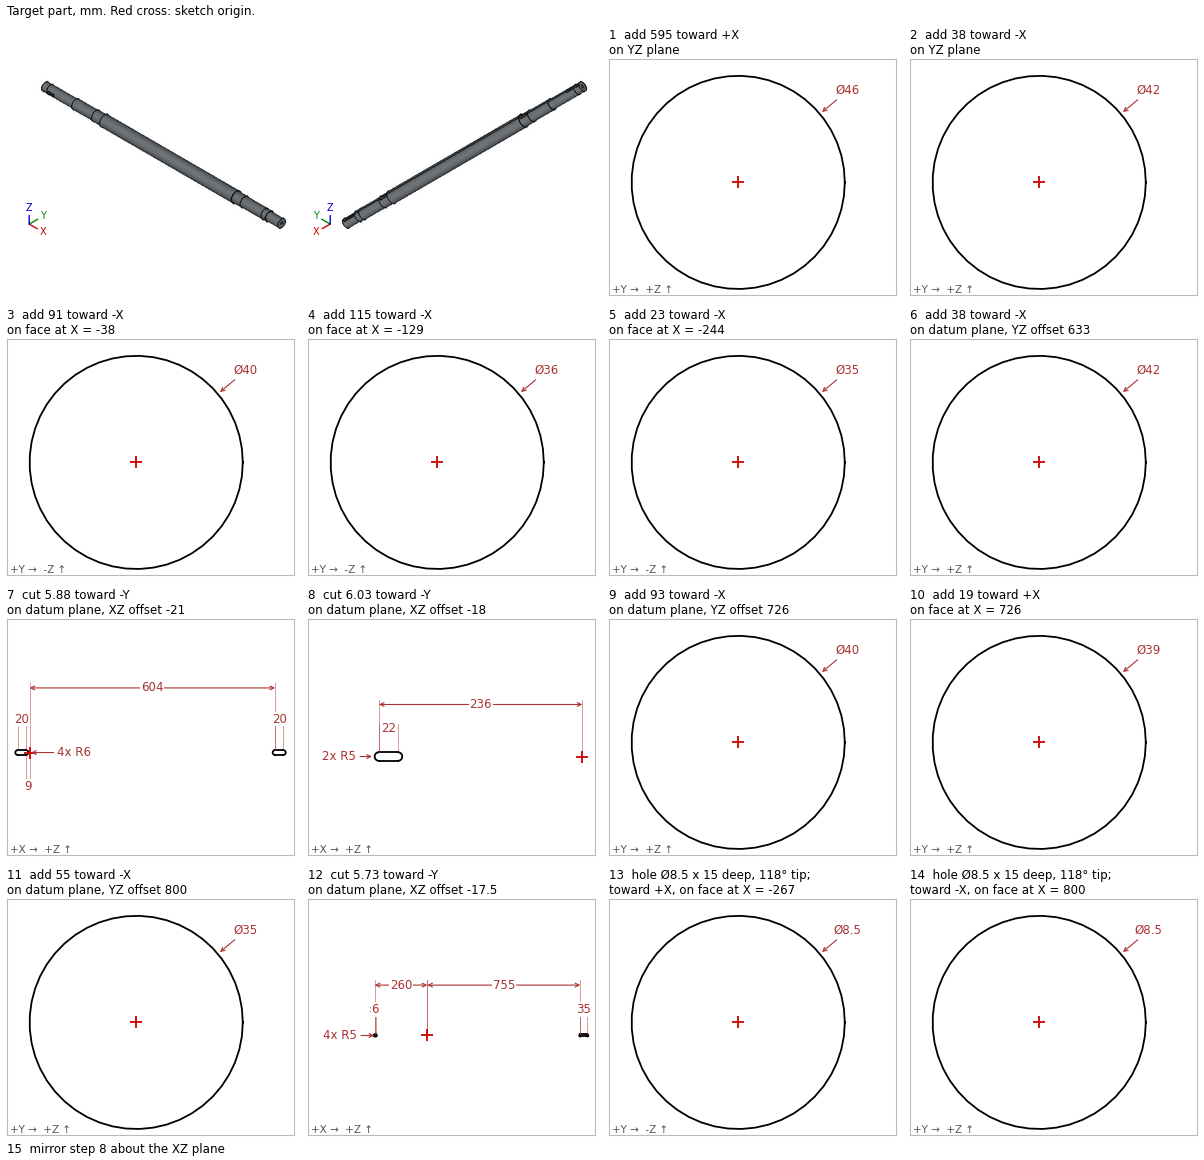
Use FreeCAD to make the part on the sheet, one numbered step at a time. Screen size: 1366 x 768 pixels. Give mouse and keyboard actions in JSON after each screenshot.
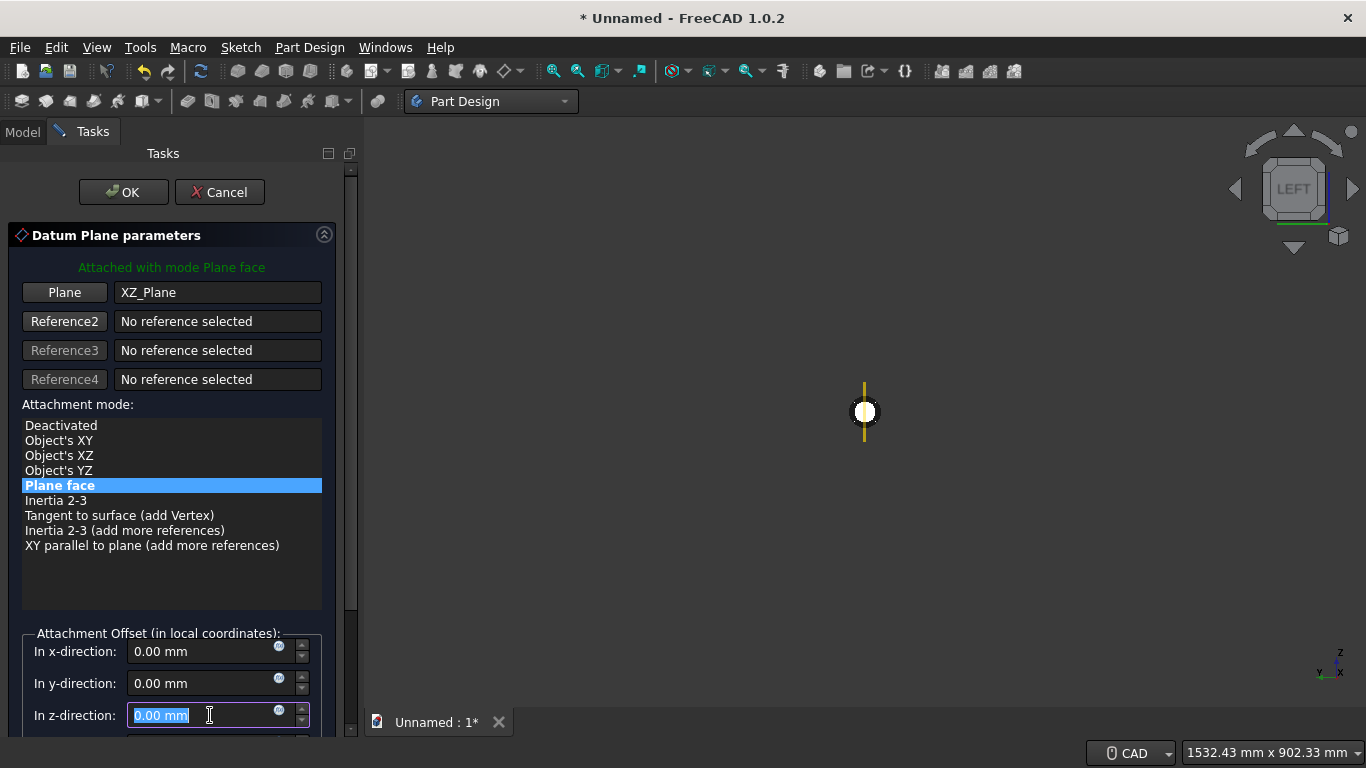
{"action": "type", "text": "-18"}
{"action": "key", "text": "Tab"}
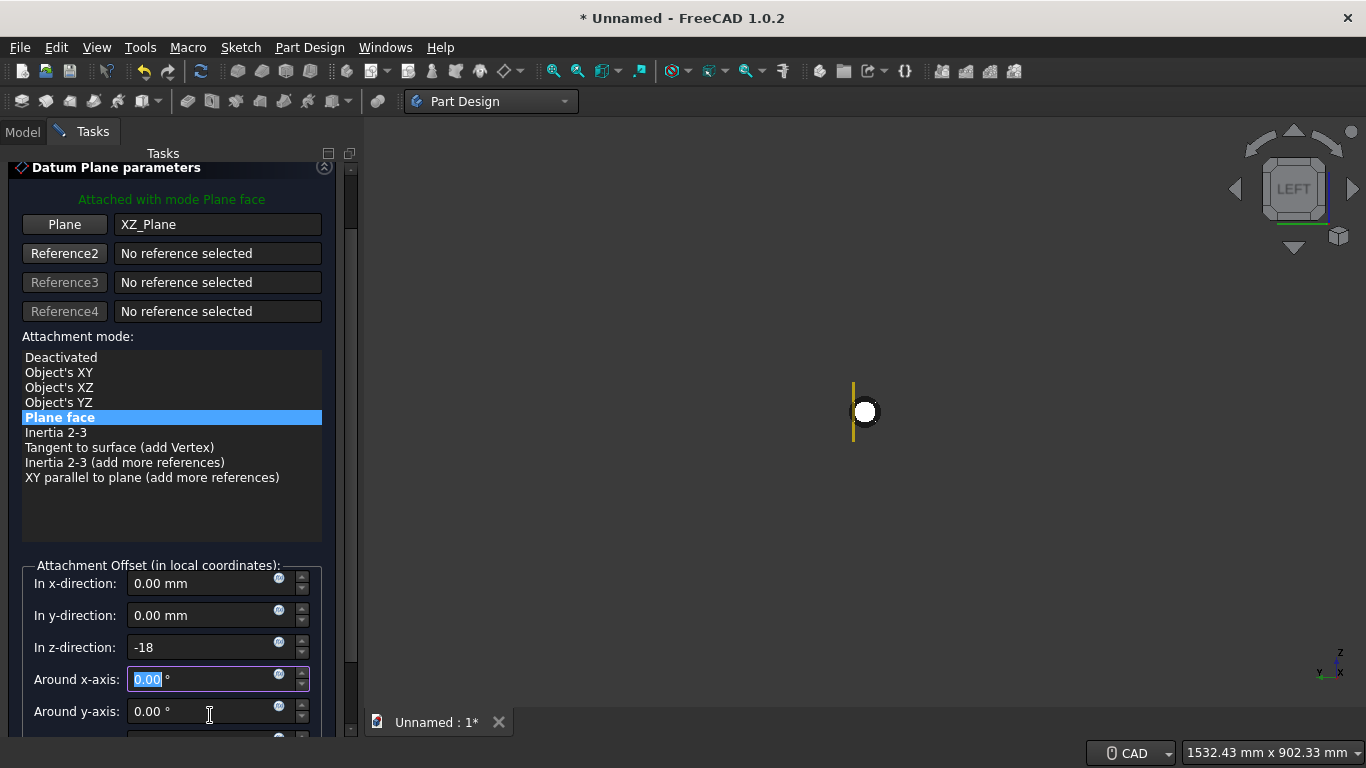
{"action": "scroll", "coordinate": [351, 450], "scroll_direction": "up", "scroll_amount": 2}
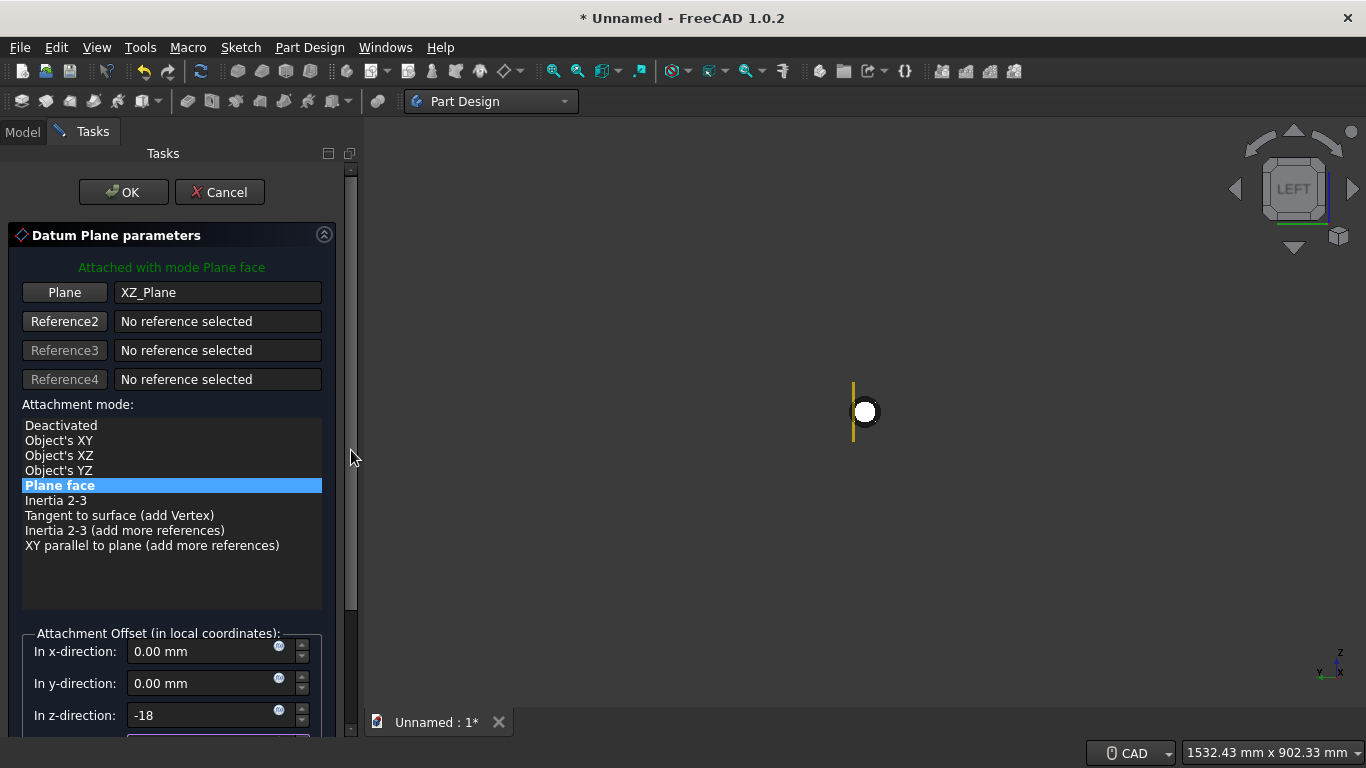
{"action": "left_click", "coordinate": [124, 192]}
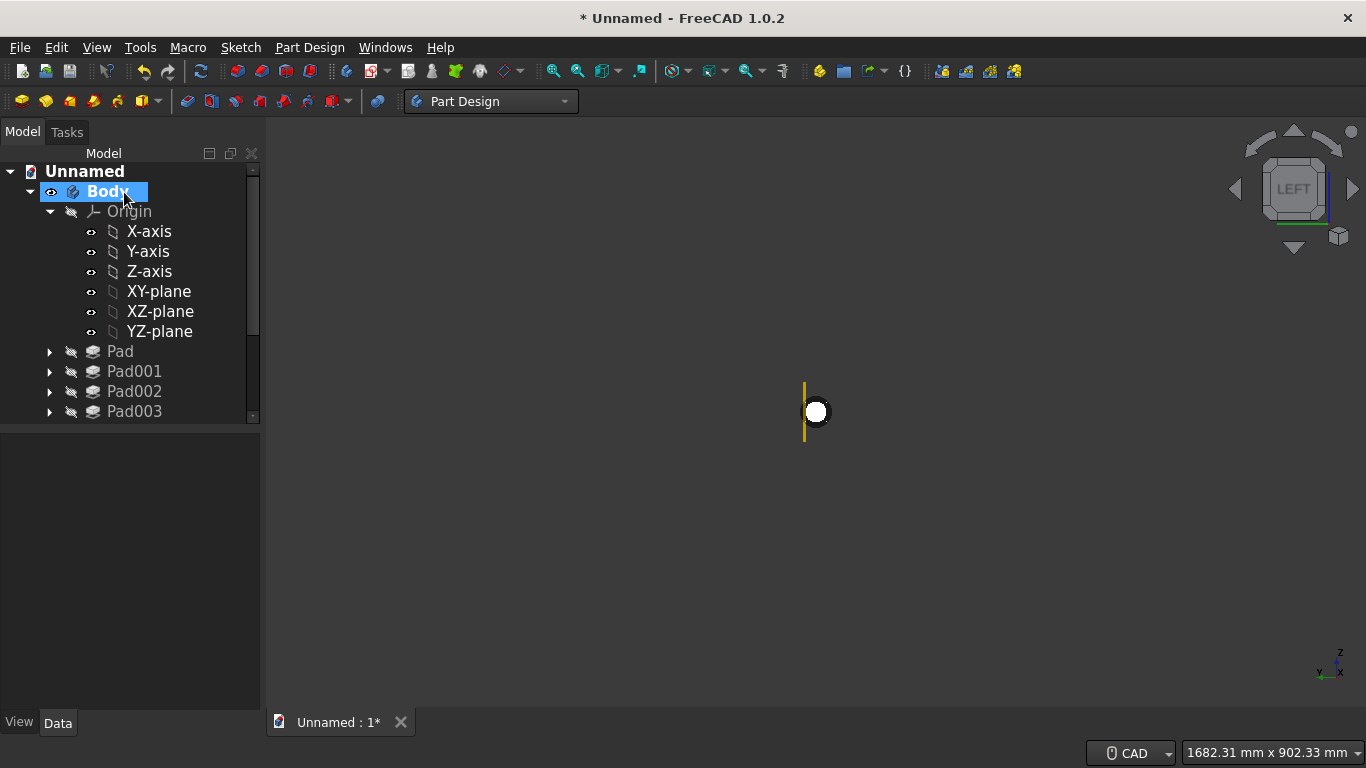
{"action": "scroll", "coordinate": [100, 287], "scroll_direction": "down", "scroll_amount": 3}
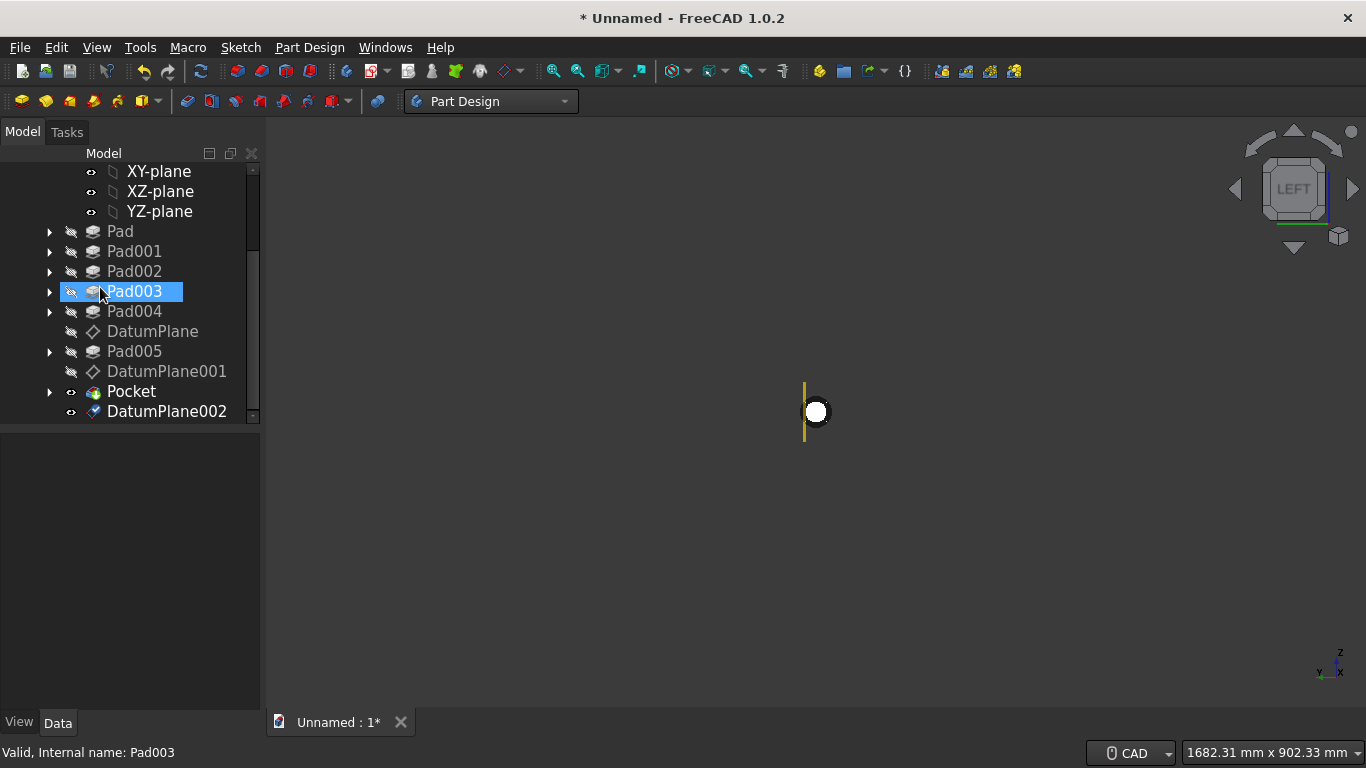
{"action": "left_click", "coordinate": [116, 412]}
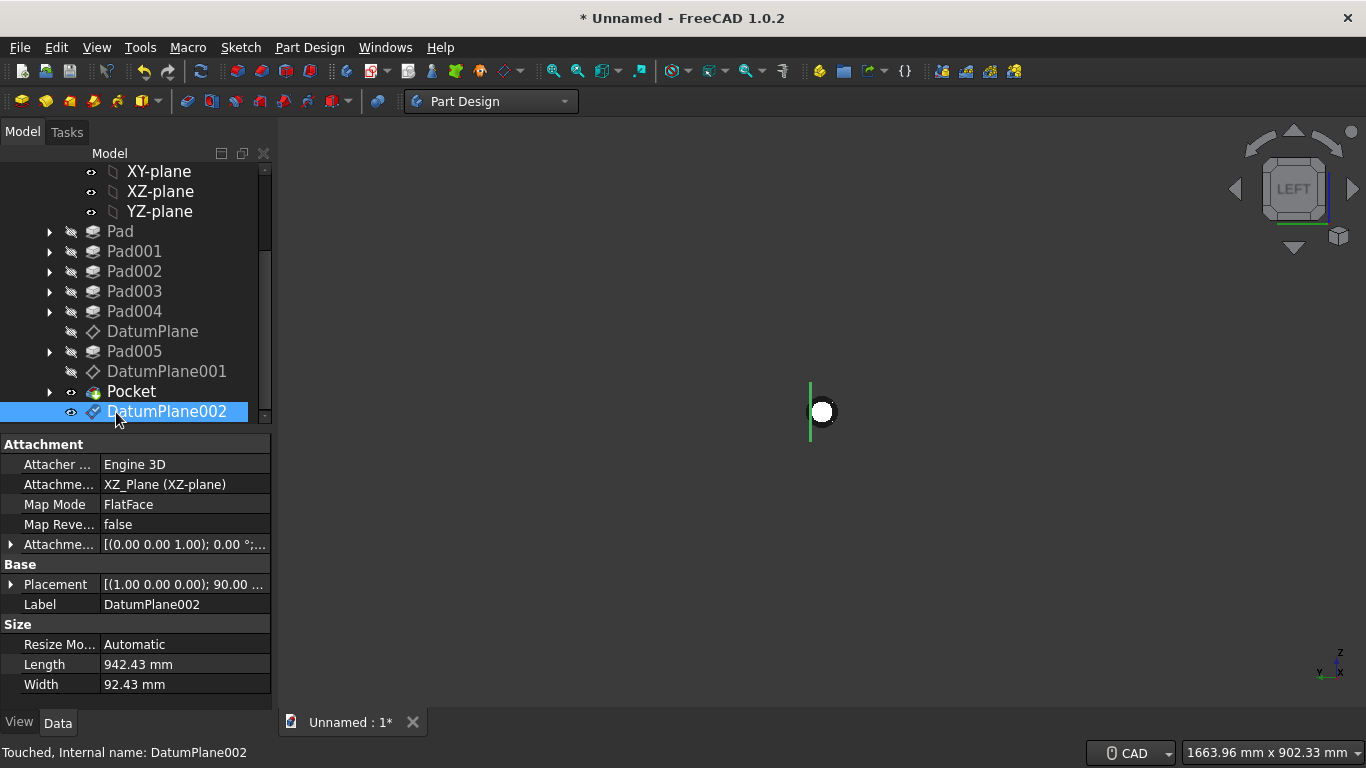
{"action": "left_click", "coordinate": [372, 72]}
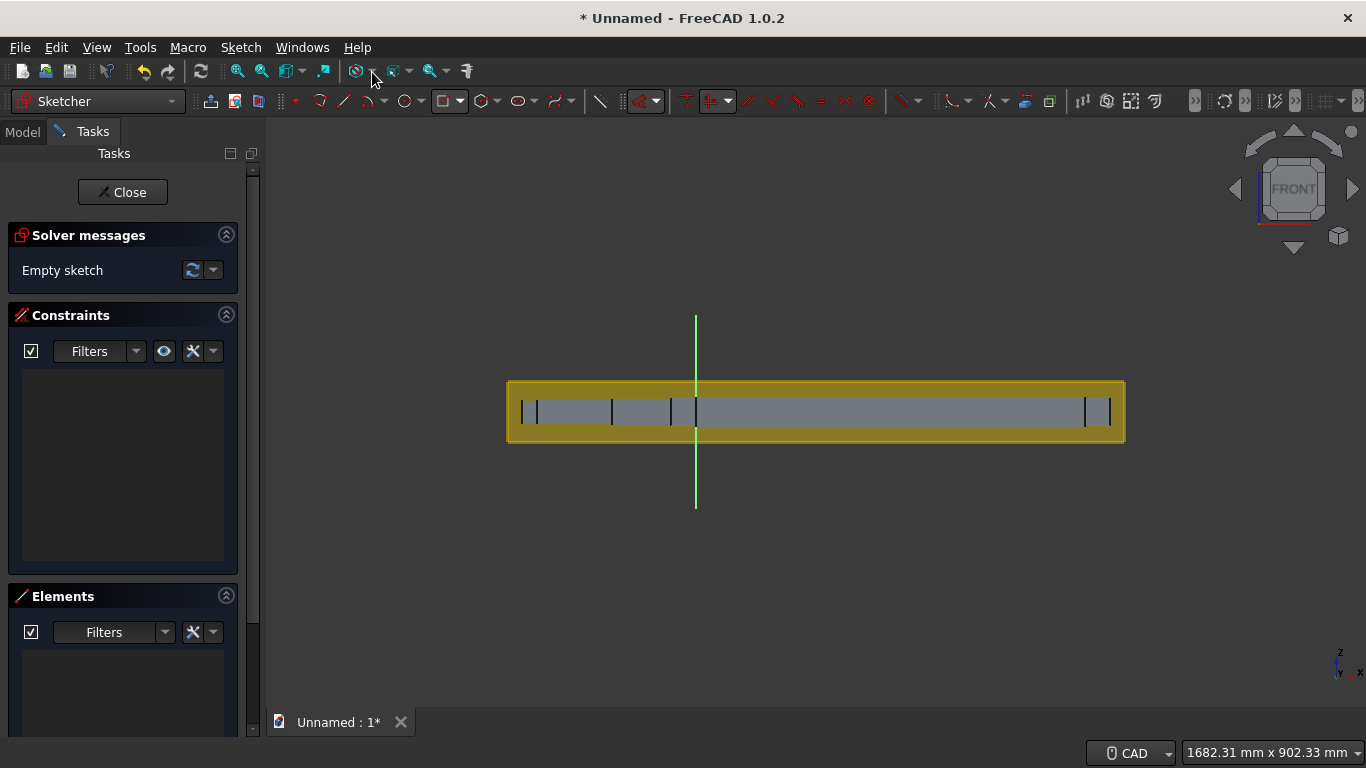
{"action": "key", "text": "q s"}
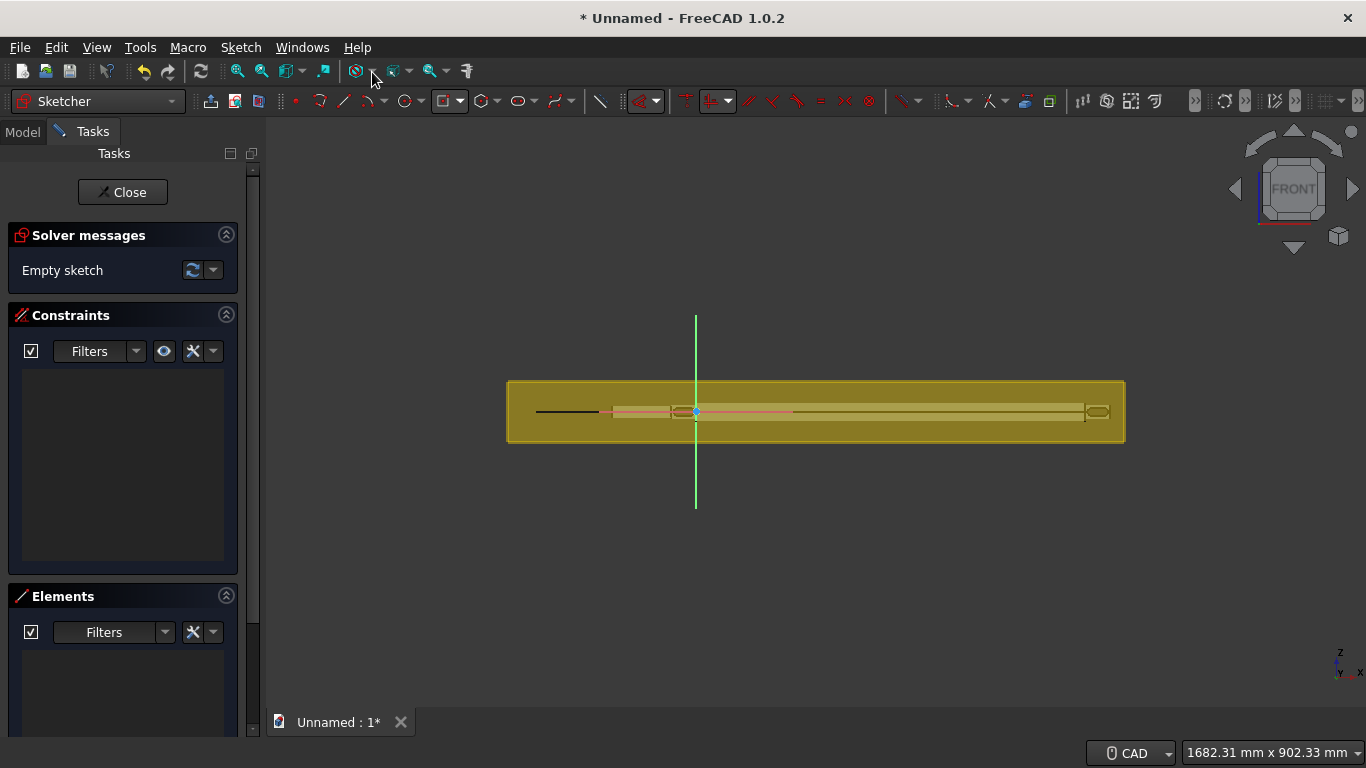
{"action": "scroll", "coordinate": [539, 412], "scroll_direction": "up", "scroll_amount": 15}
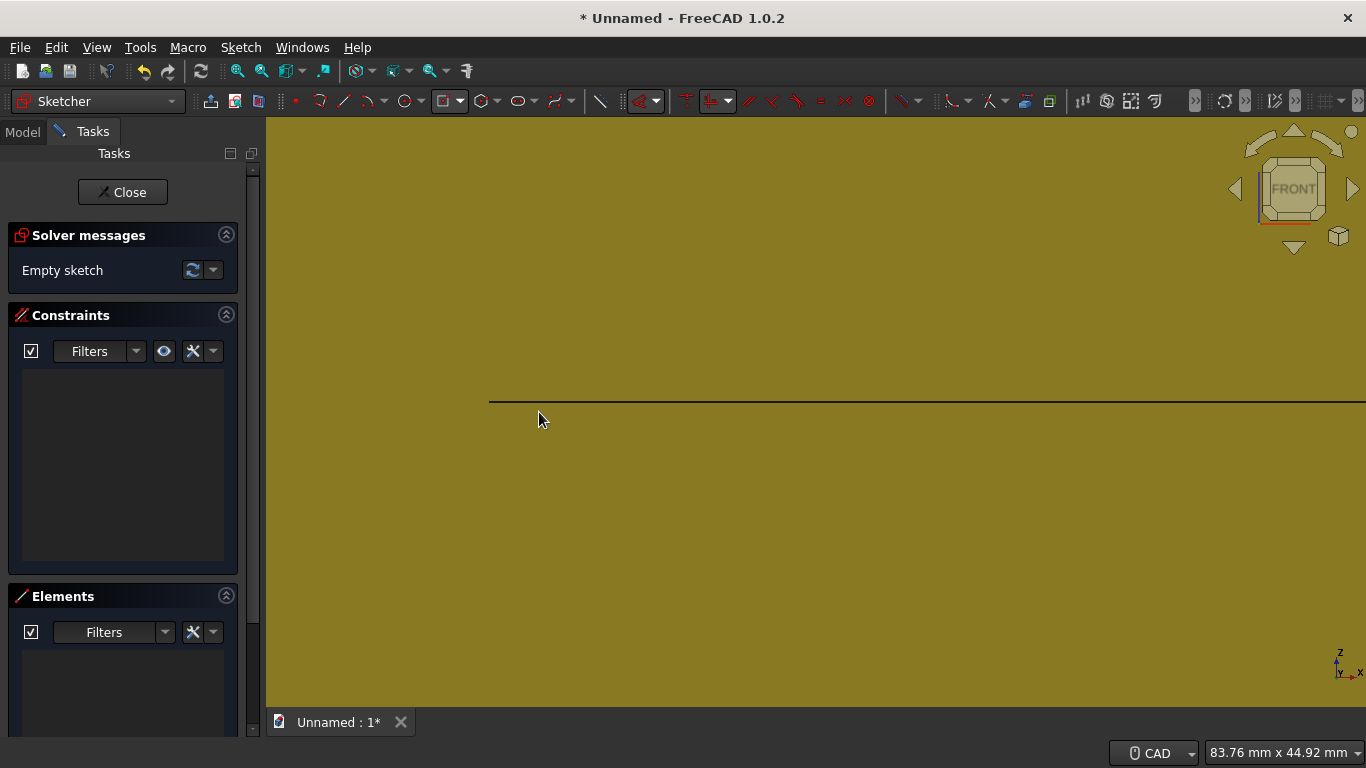
{"action": "scroll", "coordinate": [724, 383], "scroll_direction": "up", "scroll_amount": 2}